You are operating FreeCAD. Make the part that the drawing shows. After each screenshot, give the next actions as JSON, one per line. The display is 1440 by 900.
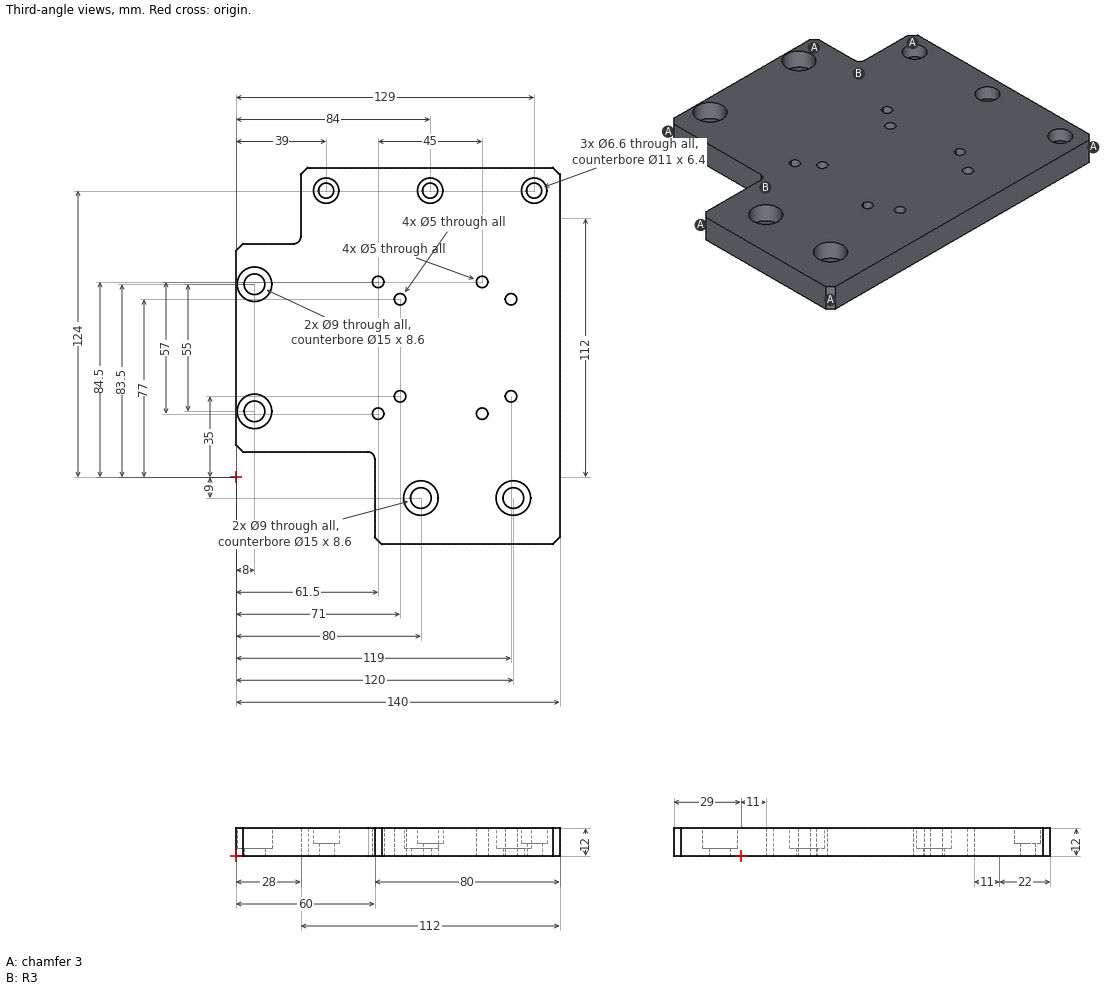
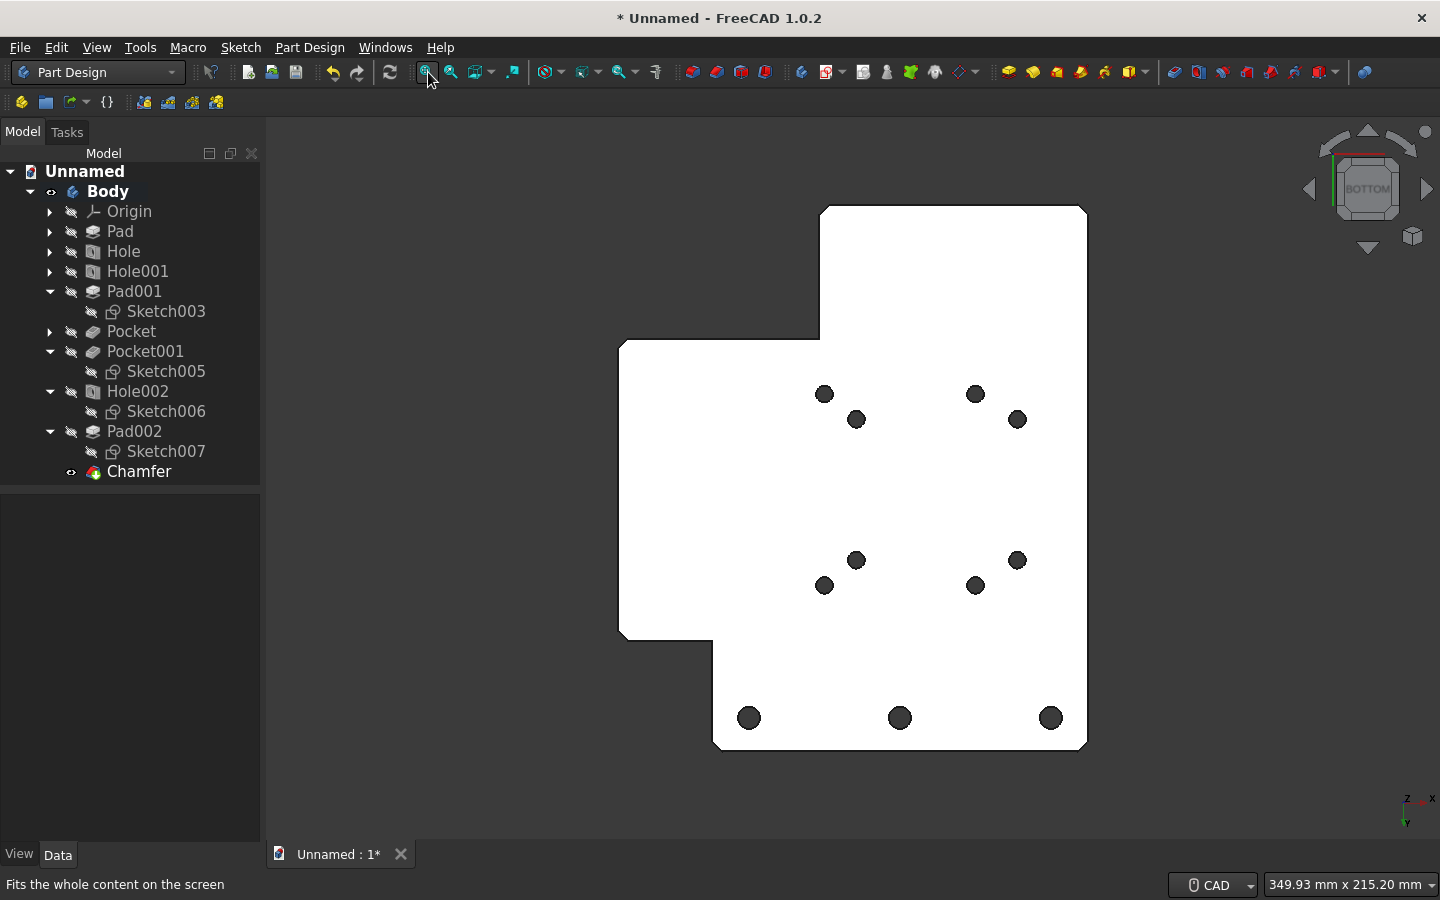
{"action": "key", "text": "4"}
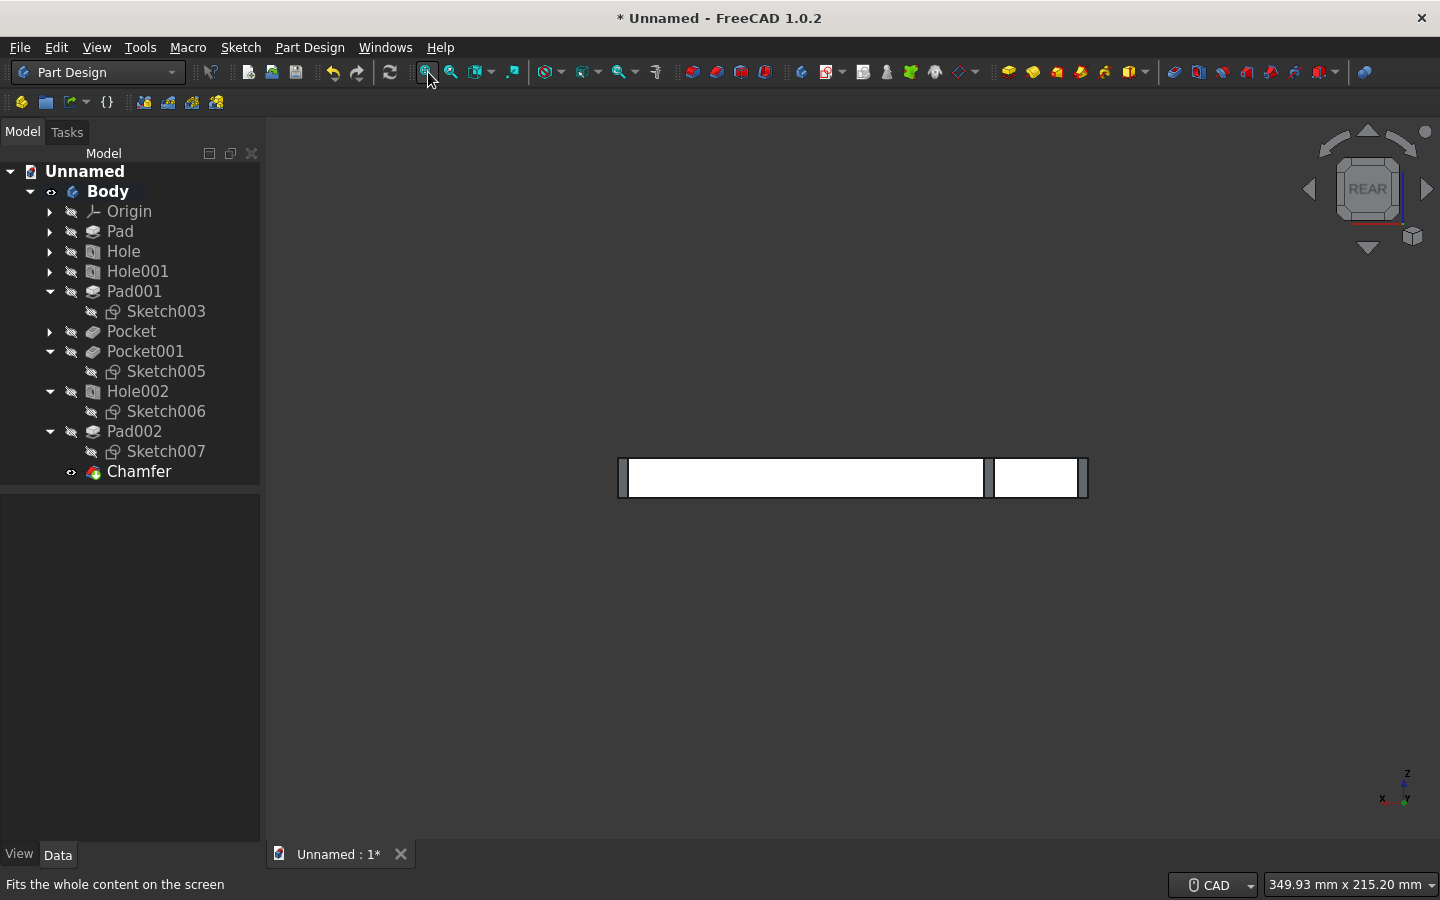
{"action": "left_click", "coordinate": [428, 72]}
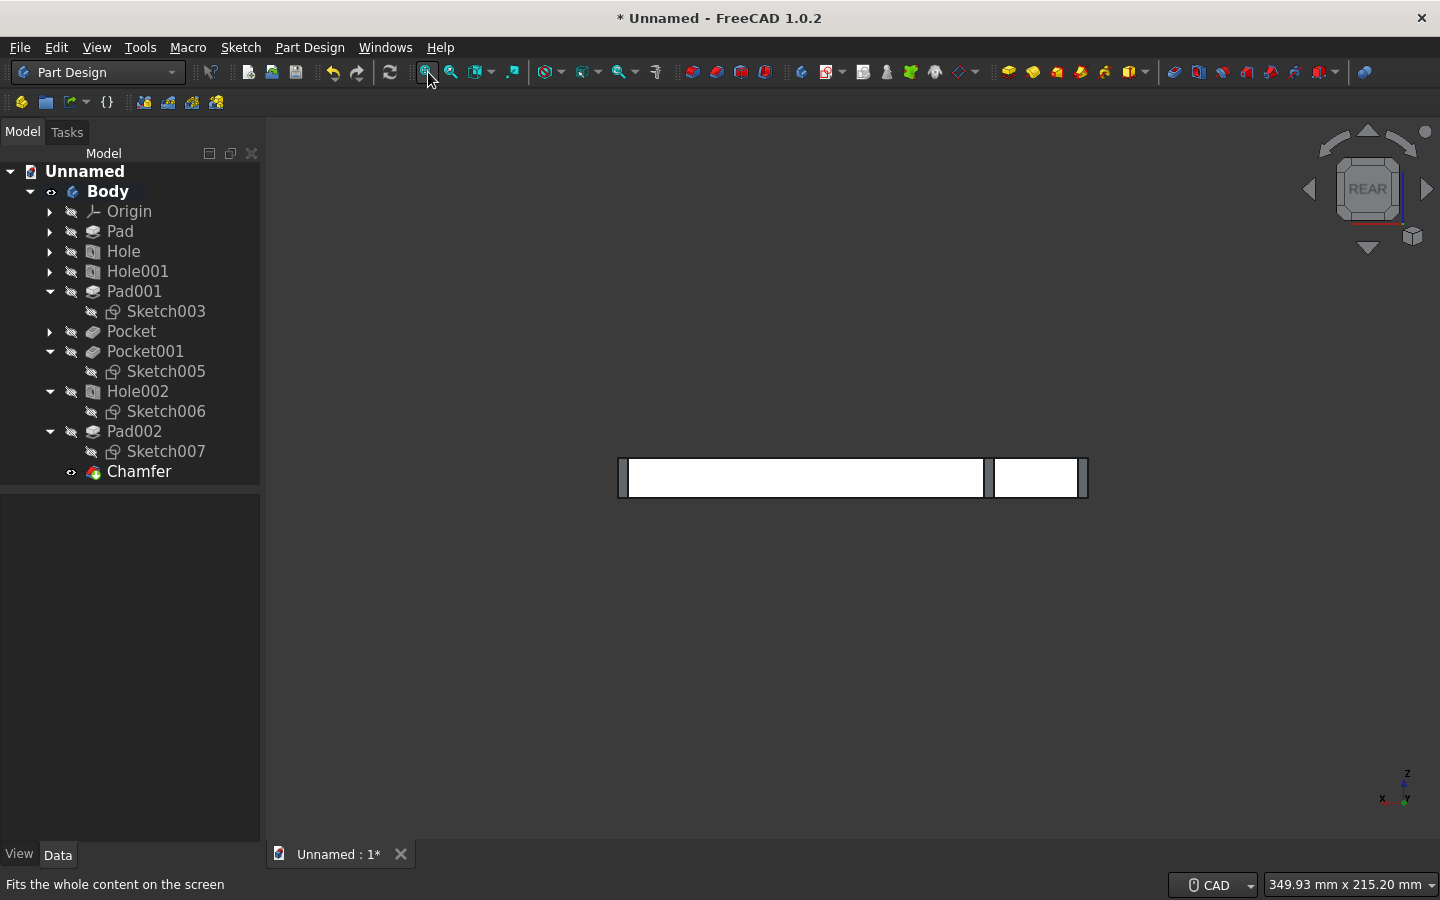
{"action": "key", "text": "6"}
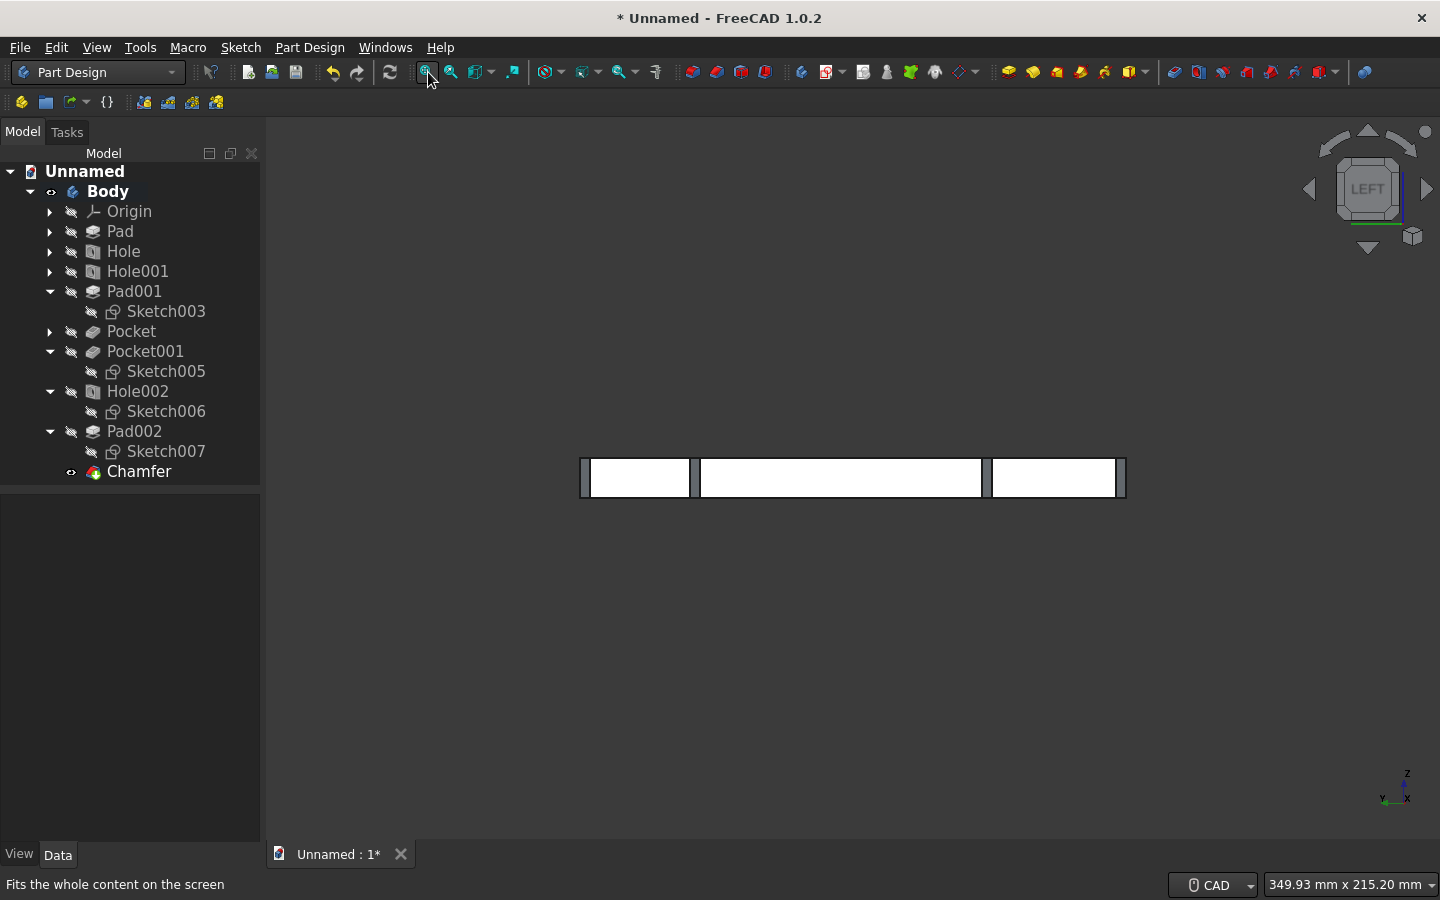
{"action": "key", "text": "v 3"}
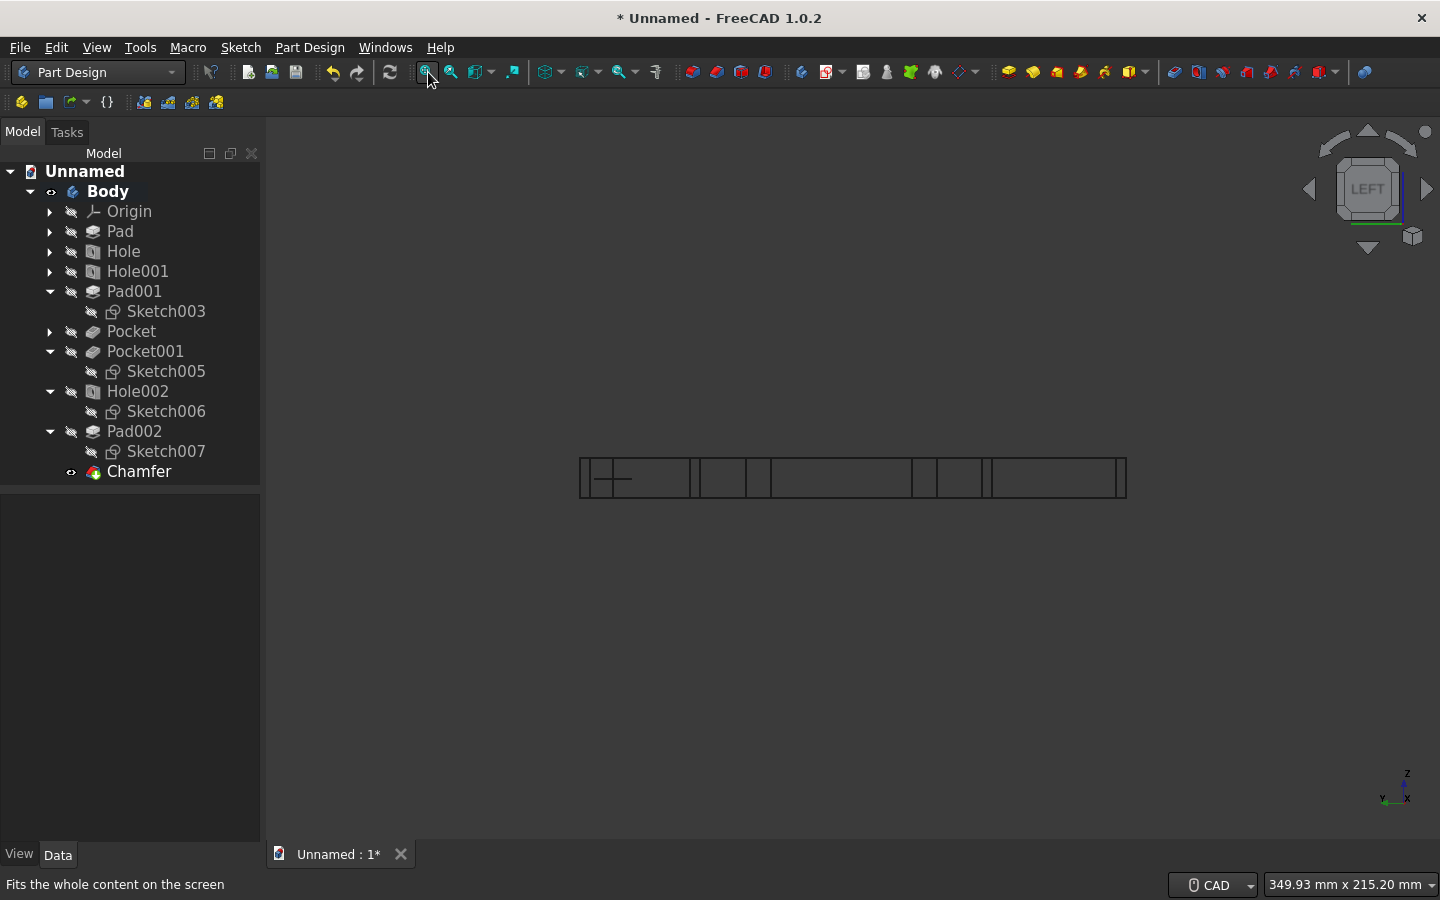
{"action": "key", "text": "0"}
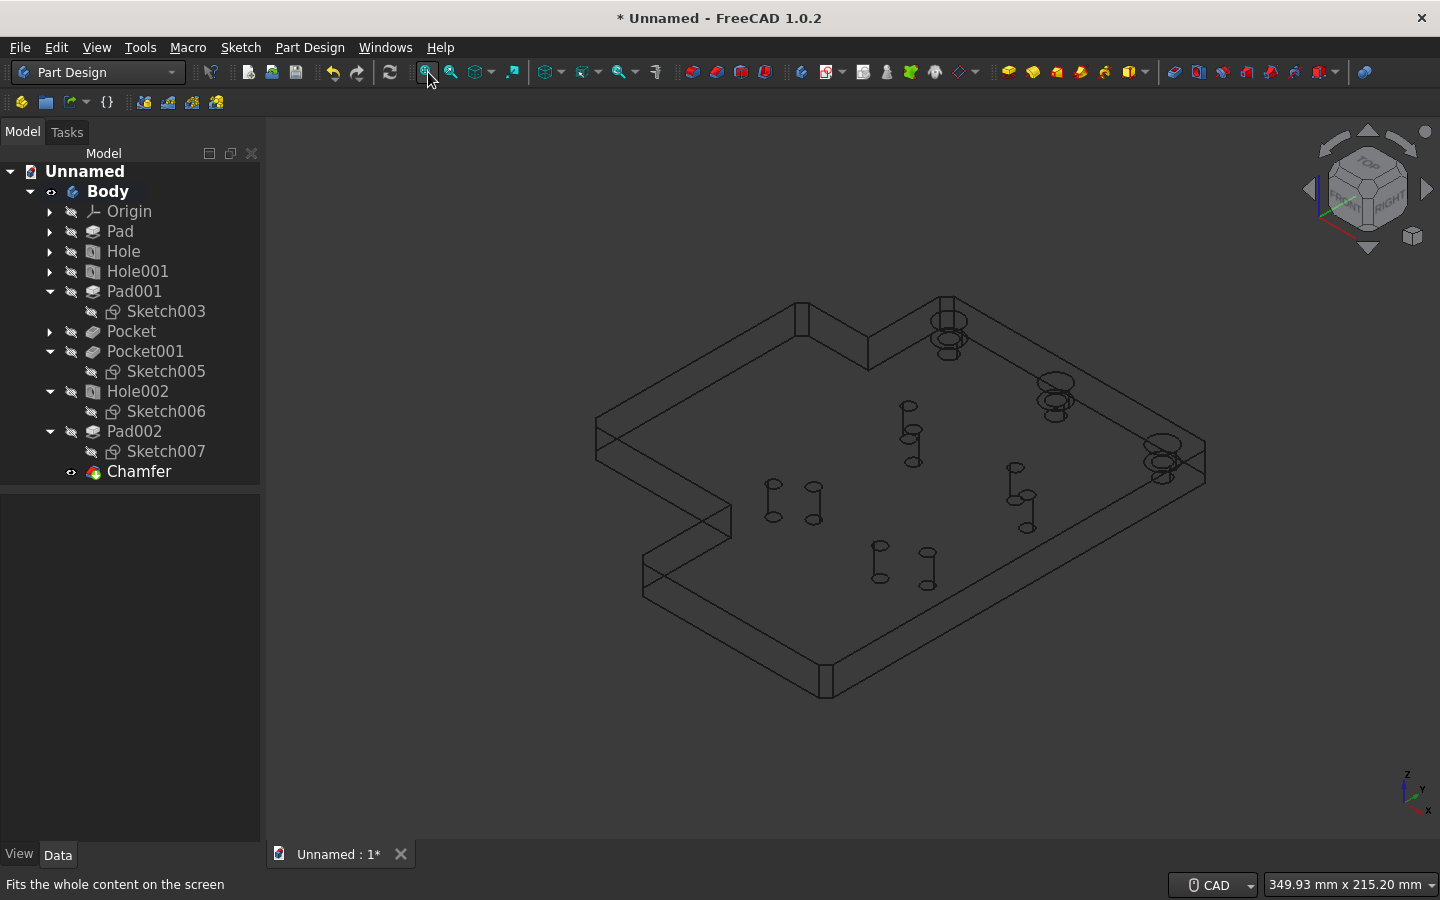
{"action": "left_click", "coordinate": [868, 353]}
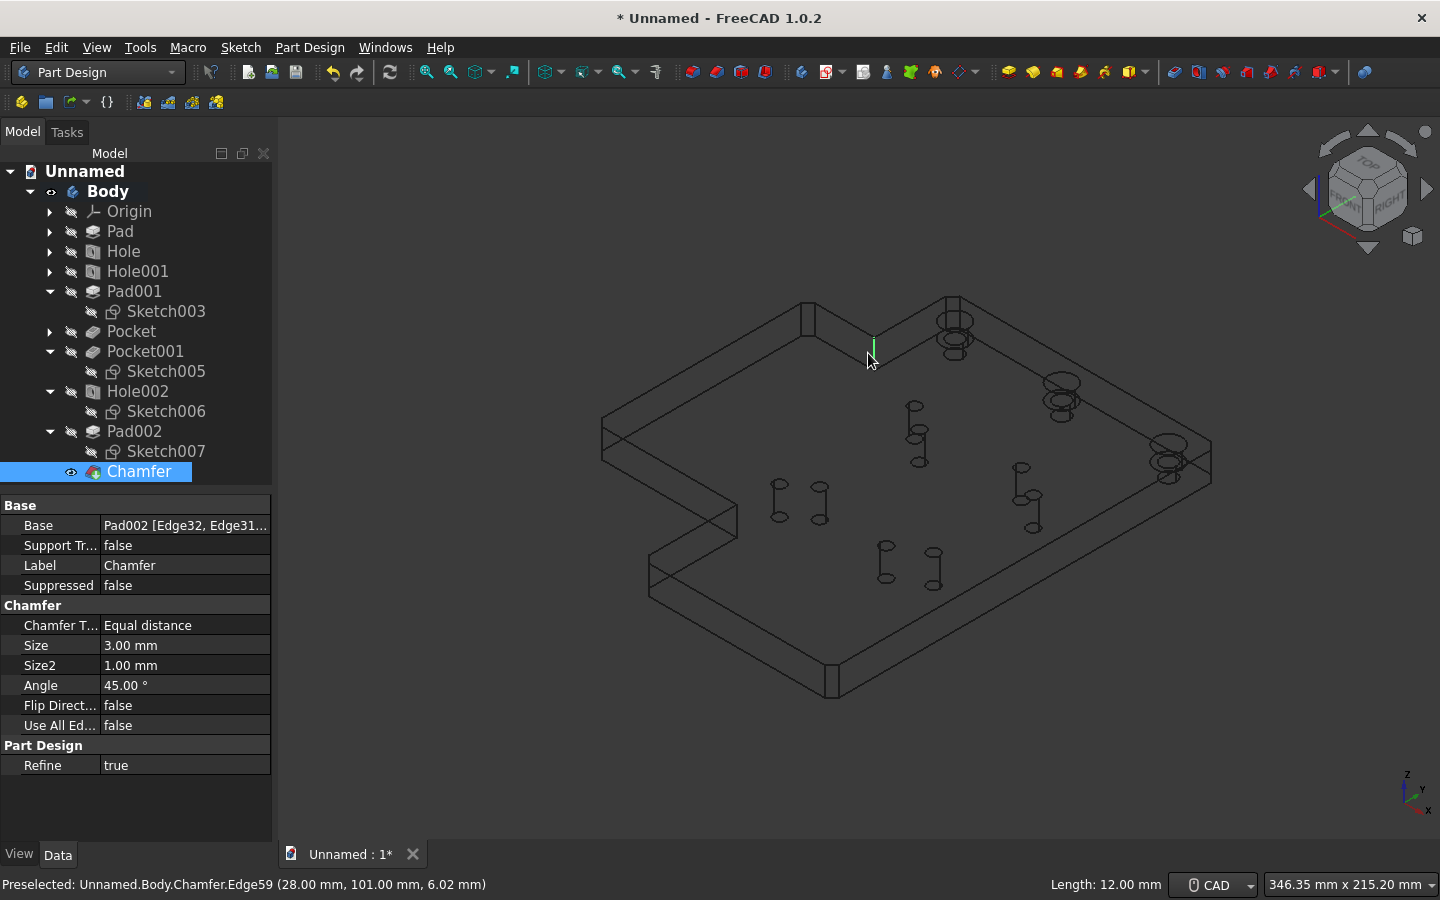
{"action": "left_click", "coordinate": [737, 520], "text": "ctrl"}